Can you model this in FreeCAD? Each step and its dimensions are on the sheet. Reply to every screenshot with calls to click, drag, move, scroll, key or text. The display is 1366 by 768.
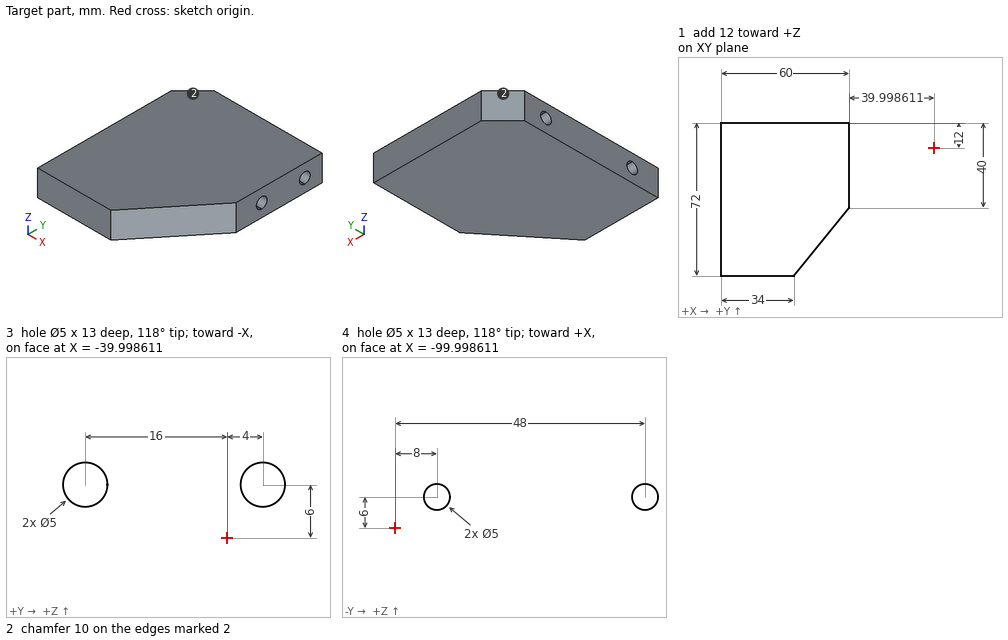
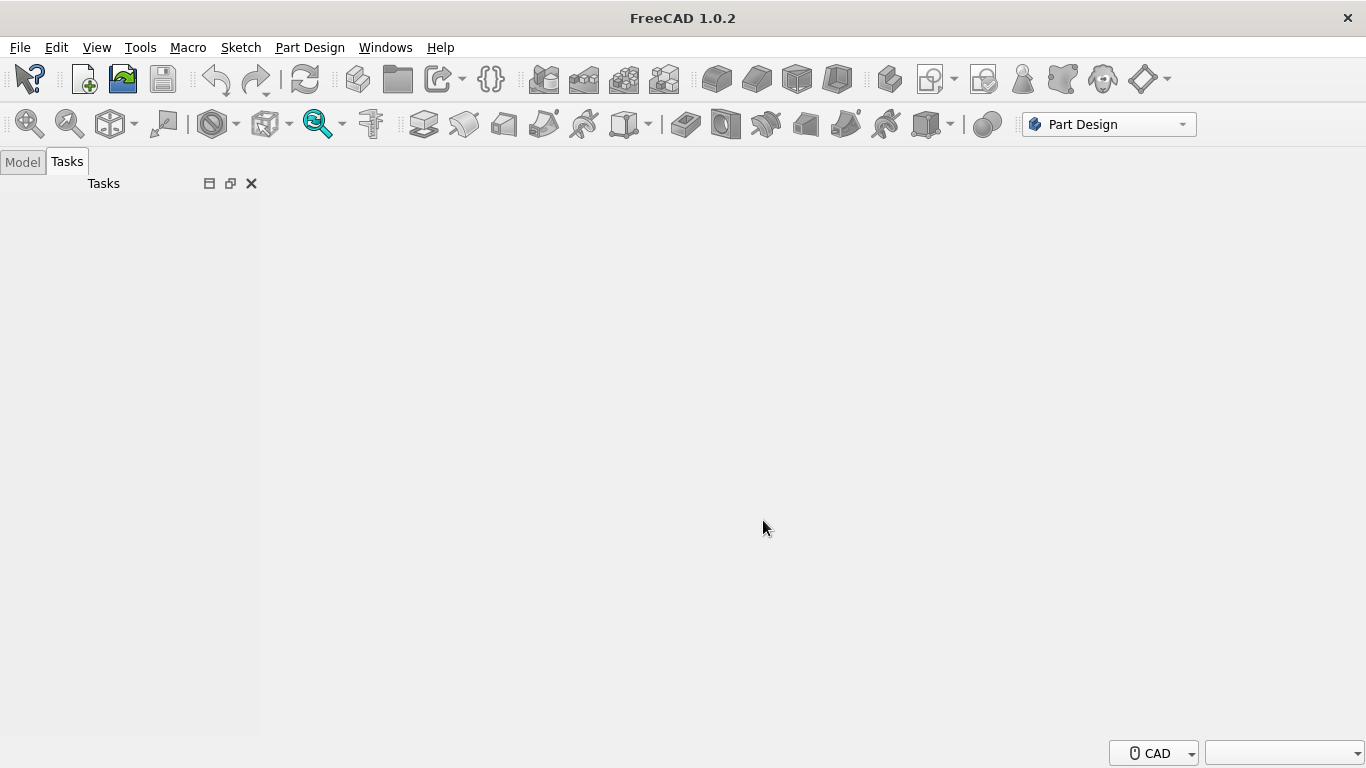
click(84, 80)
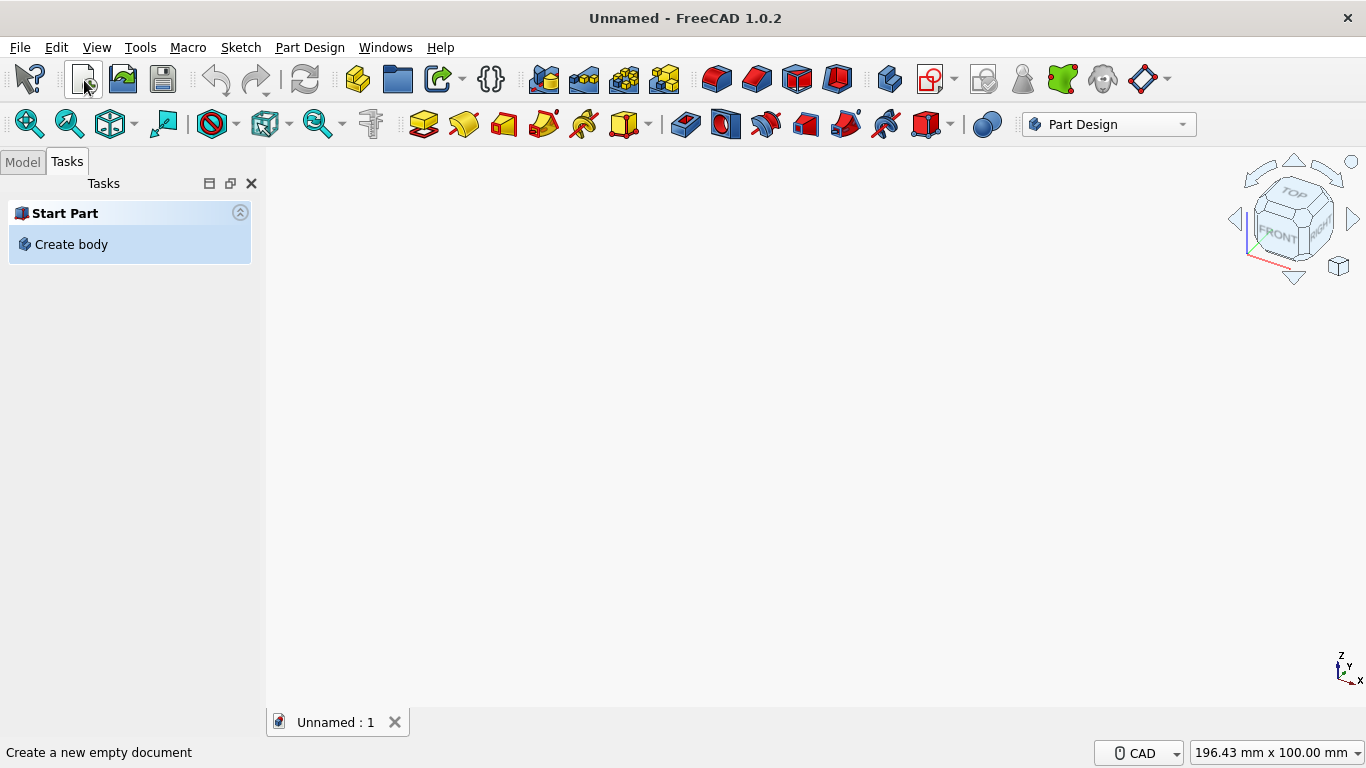
click(930, 80)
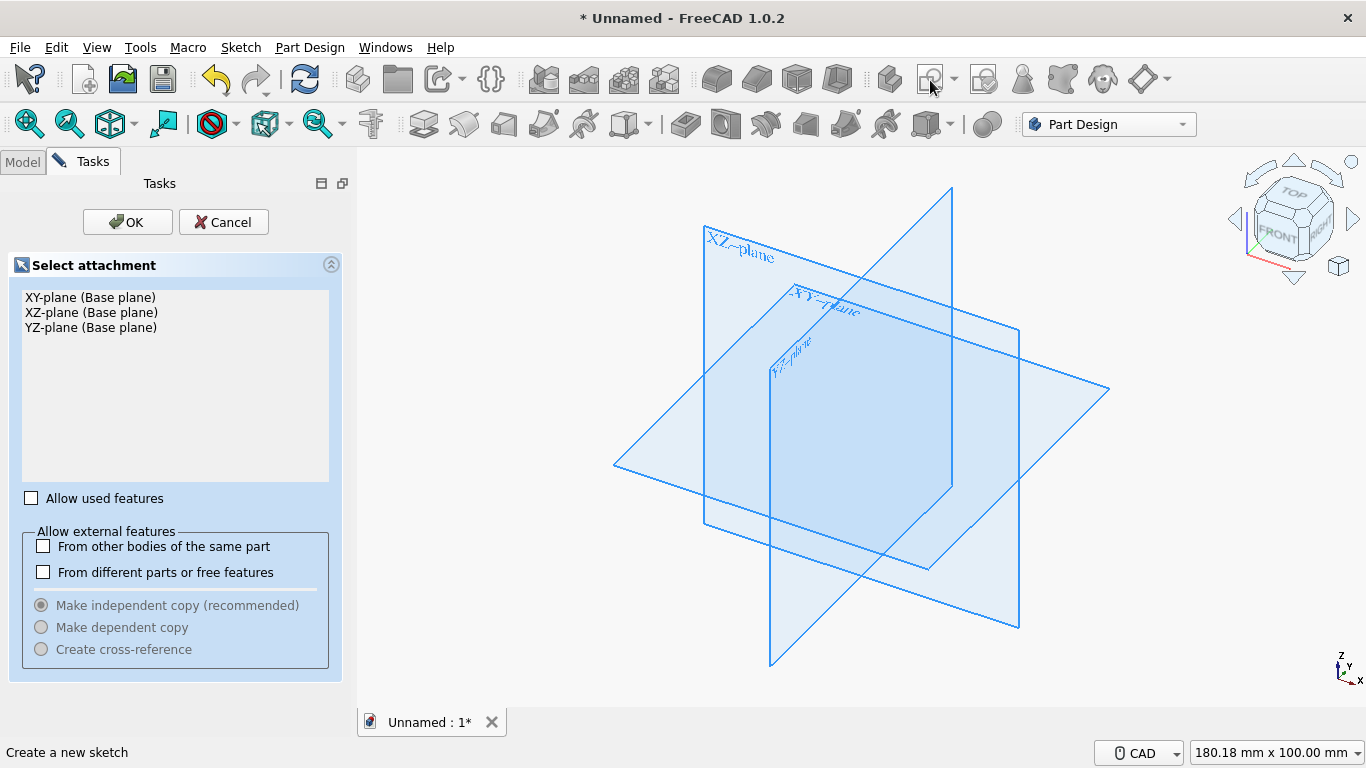
click(82, 298)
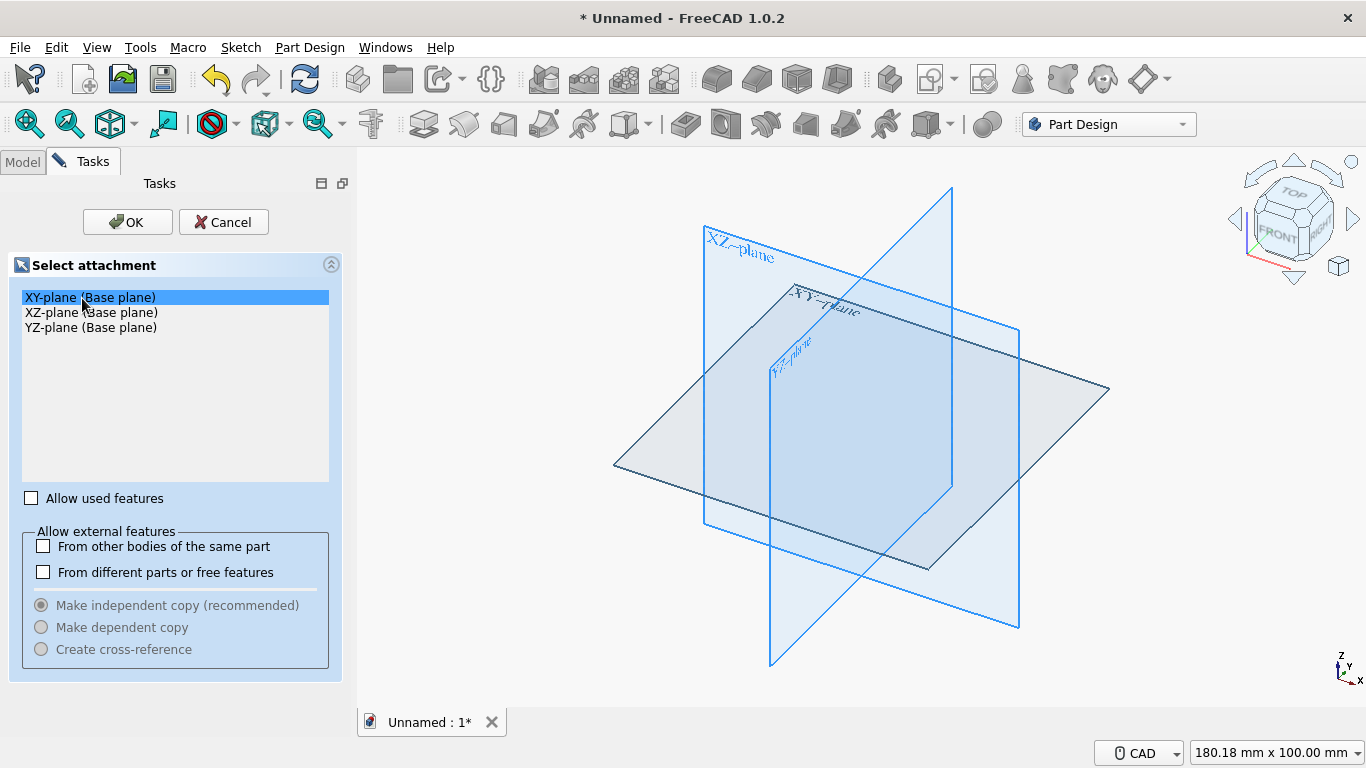
click(128, 222)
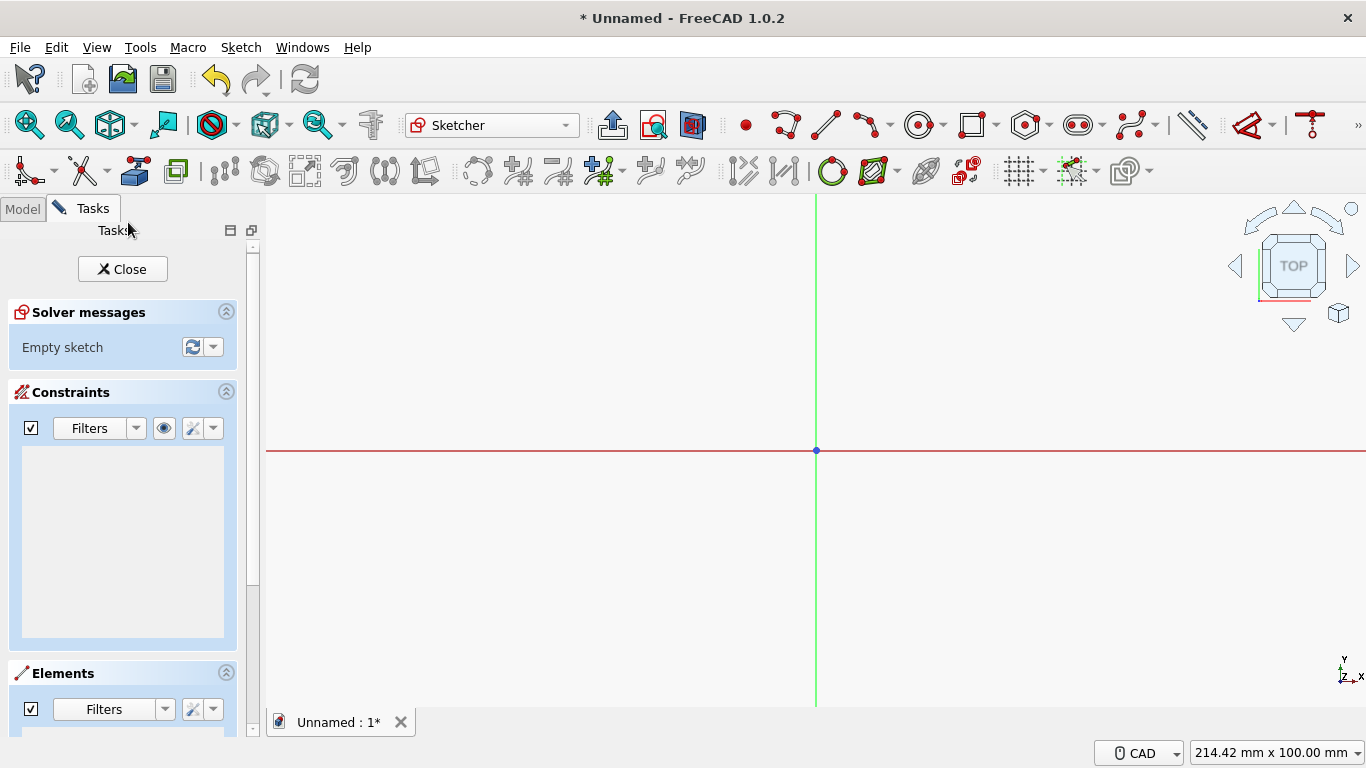
scroll(1130, 222, down, 2)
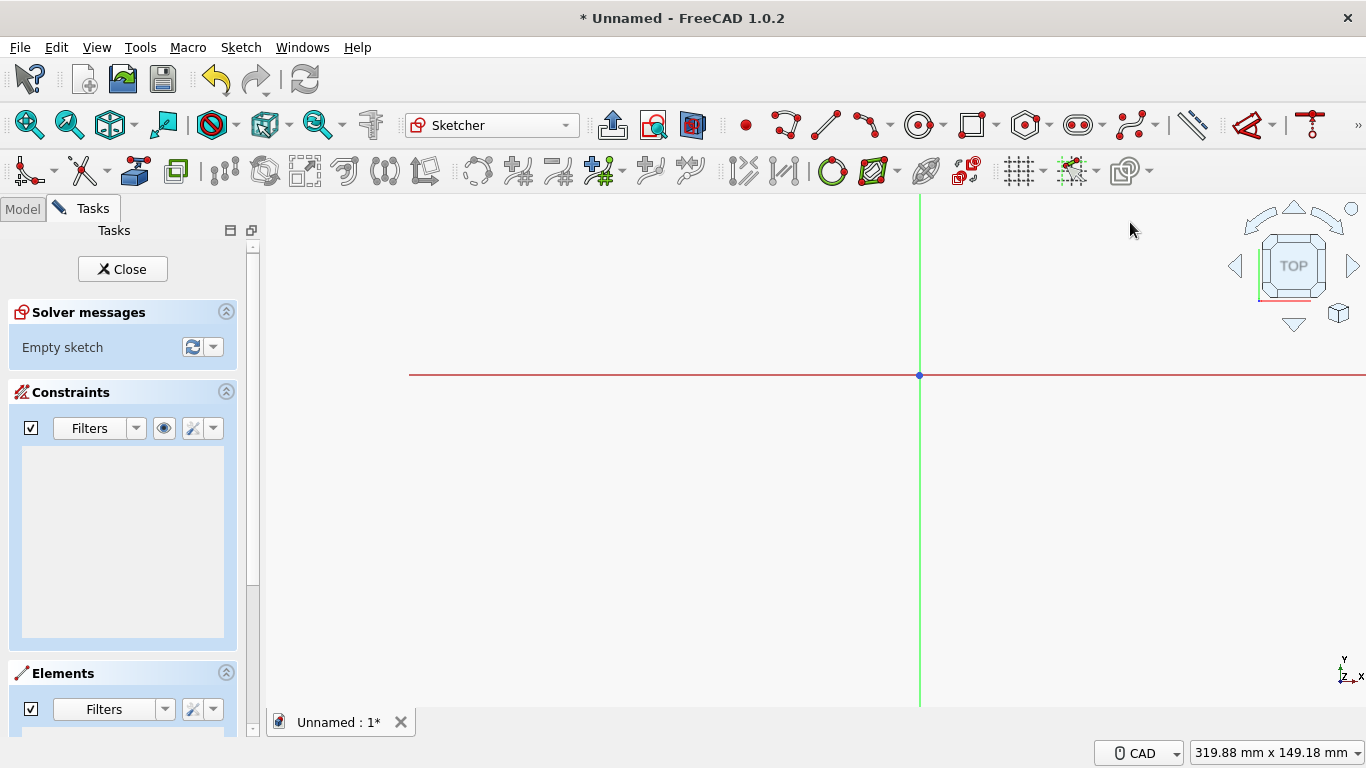
click(786, 126)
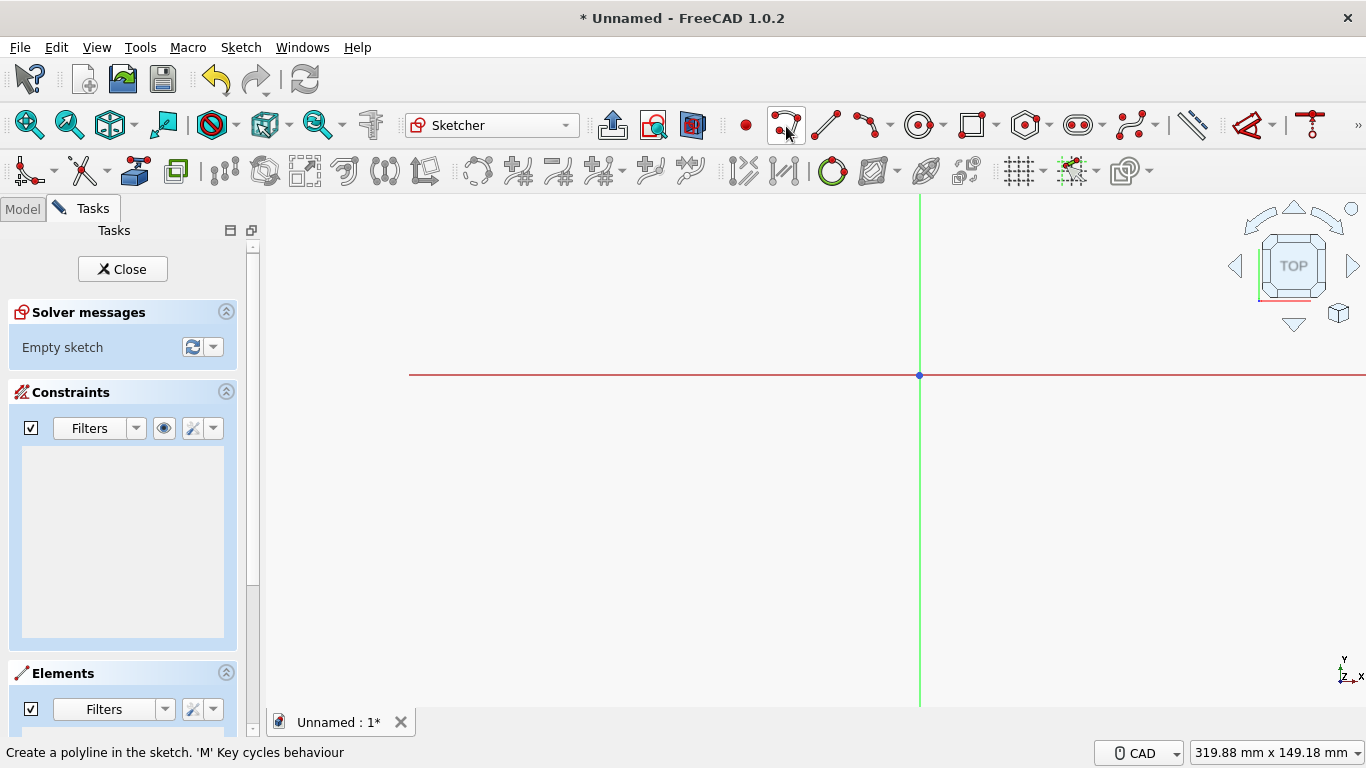
click(782, 334)
click(576, 334)
click(576, 582)
click(693, 582)
click(782, 471)
click(782, 335)
key(Escape)
key(Escape)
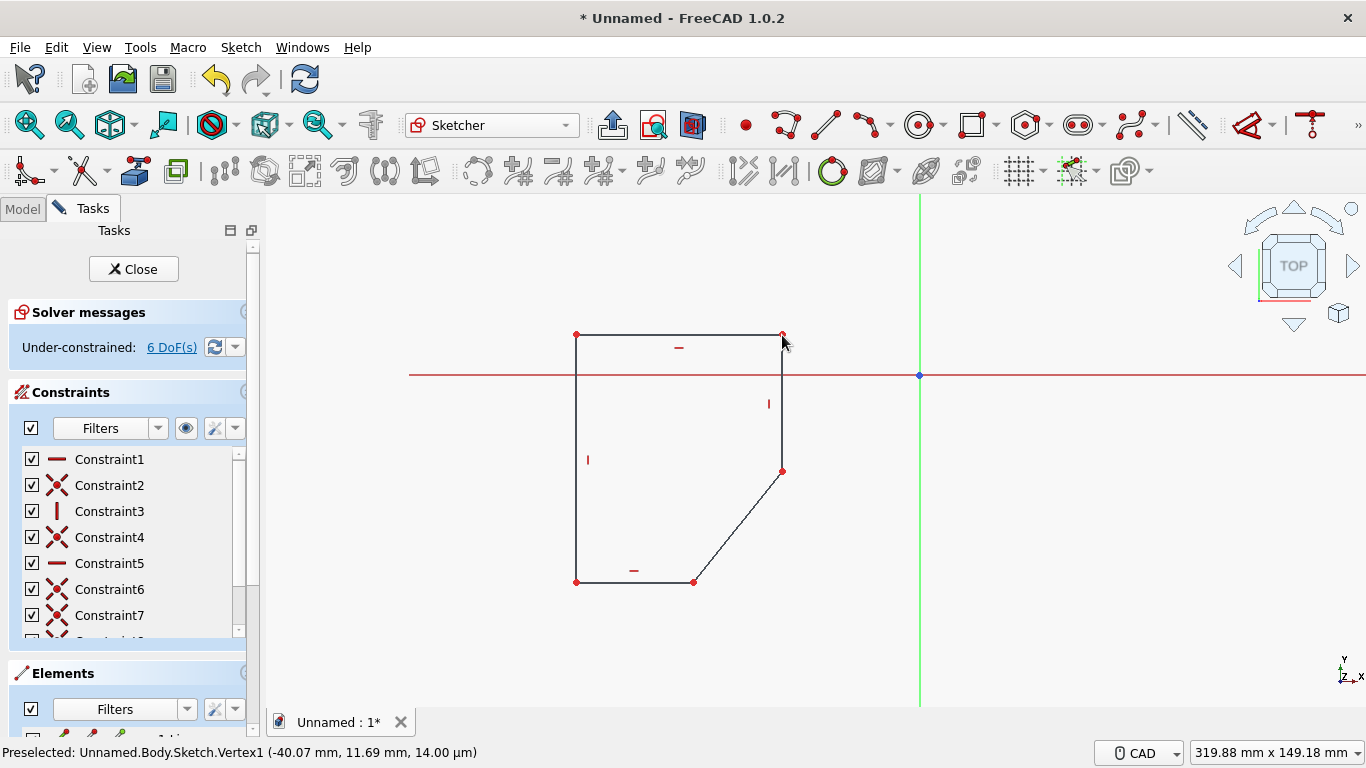
click(720, 335)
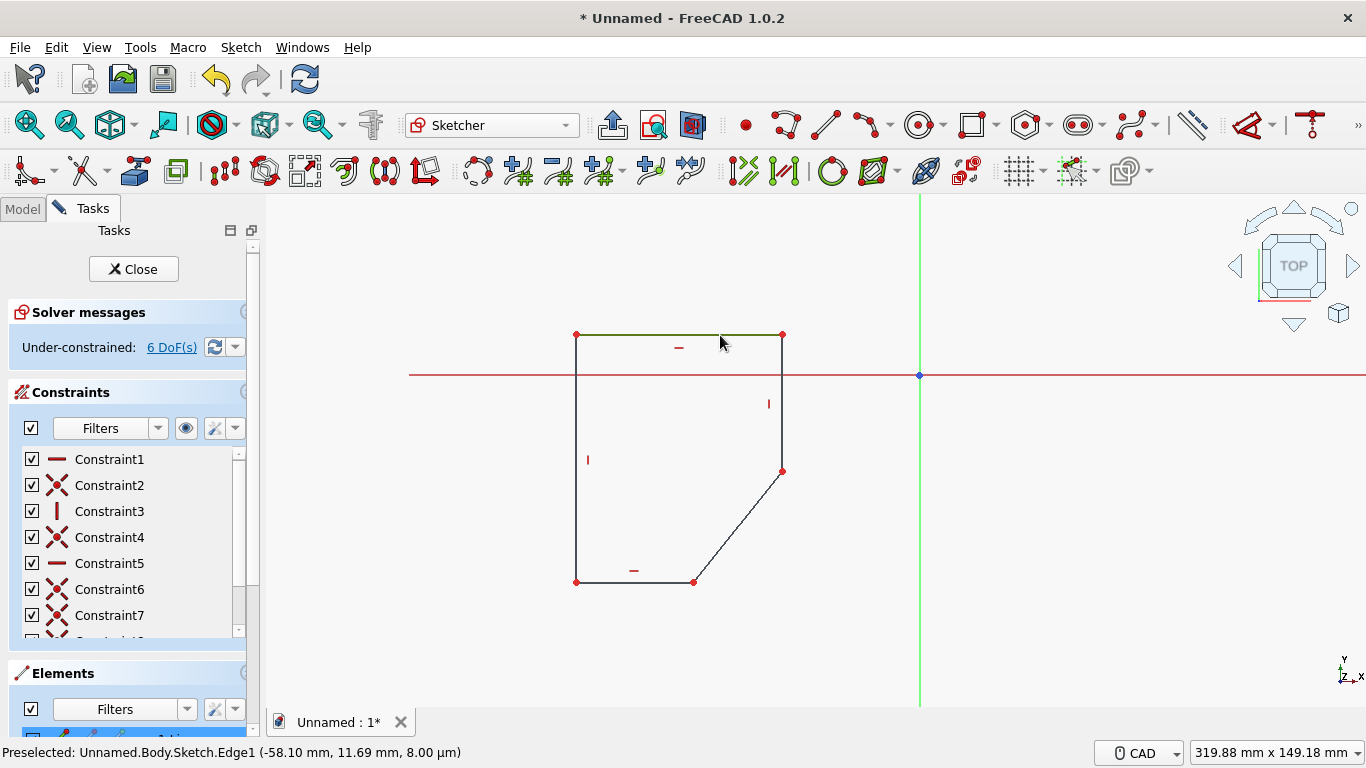
click(1274, 126)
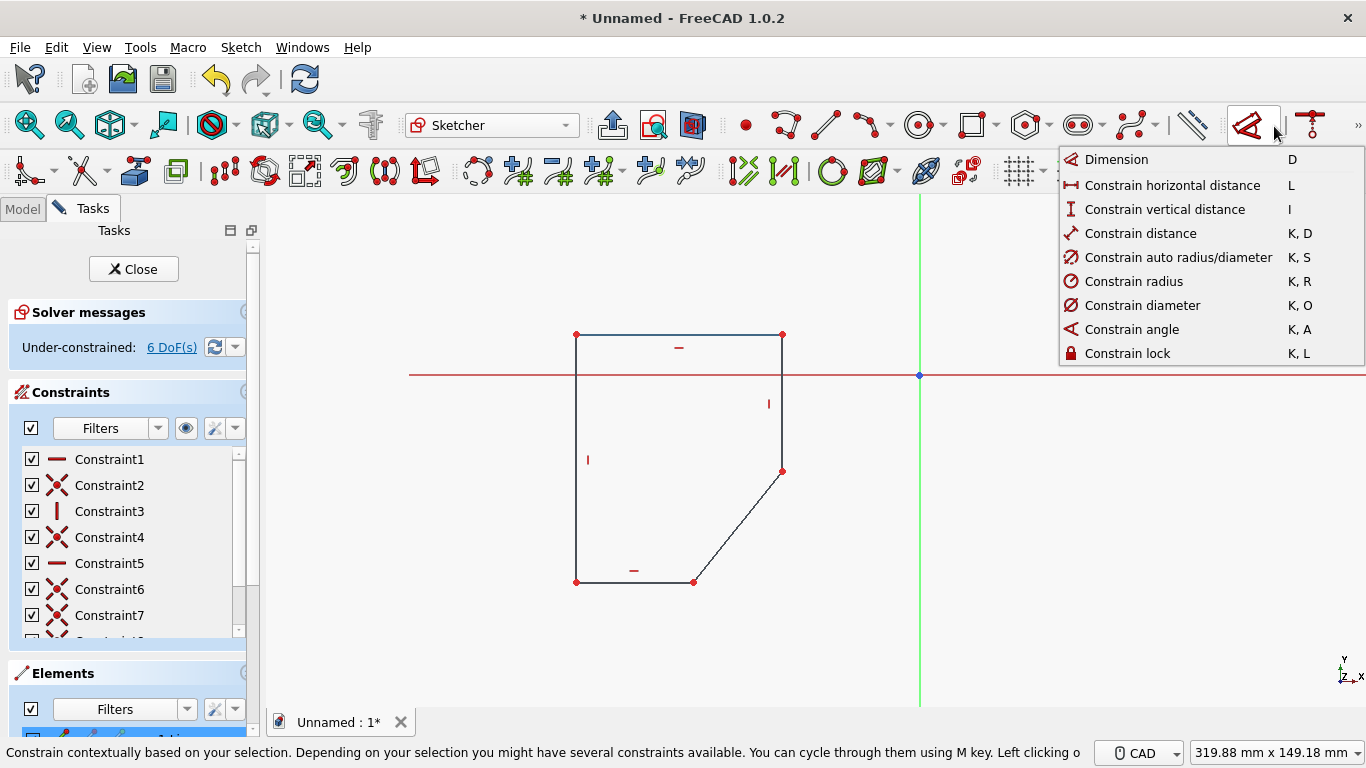
click(1212, 185)